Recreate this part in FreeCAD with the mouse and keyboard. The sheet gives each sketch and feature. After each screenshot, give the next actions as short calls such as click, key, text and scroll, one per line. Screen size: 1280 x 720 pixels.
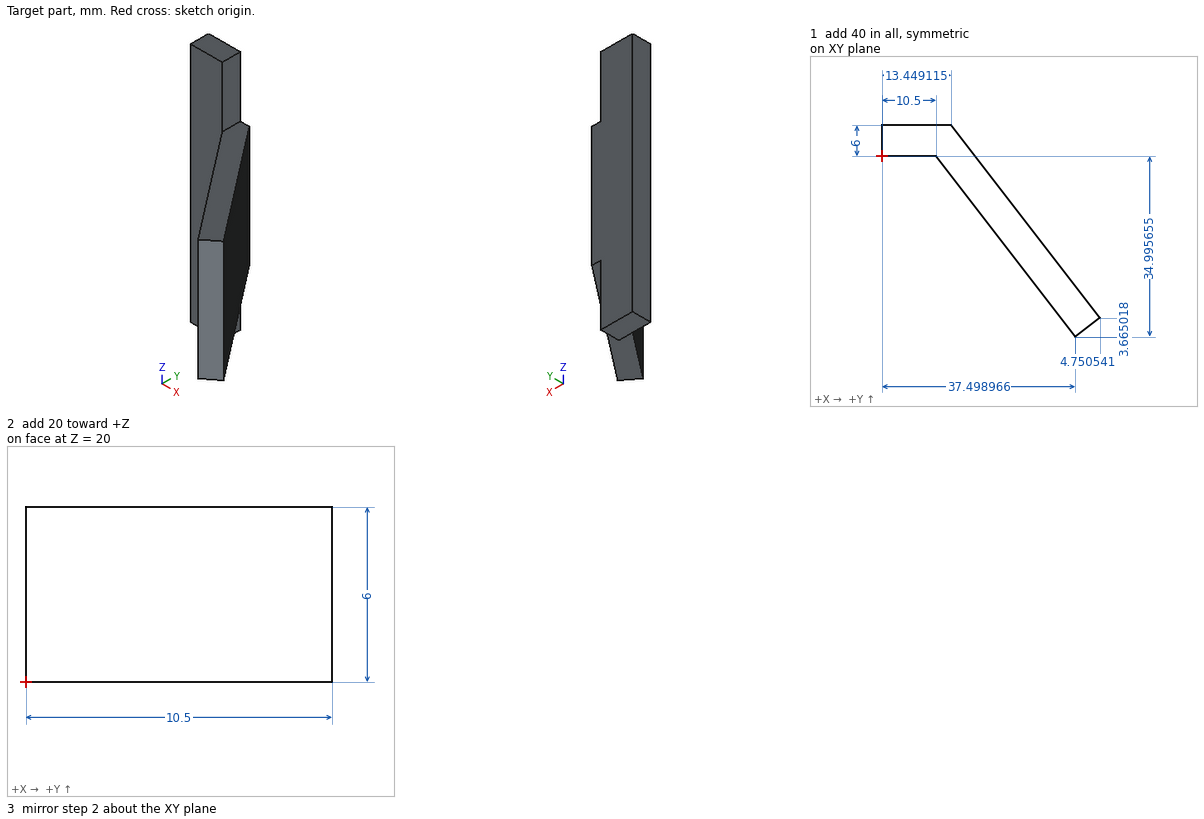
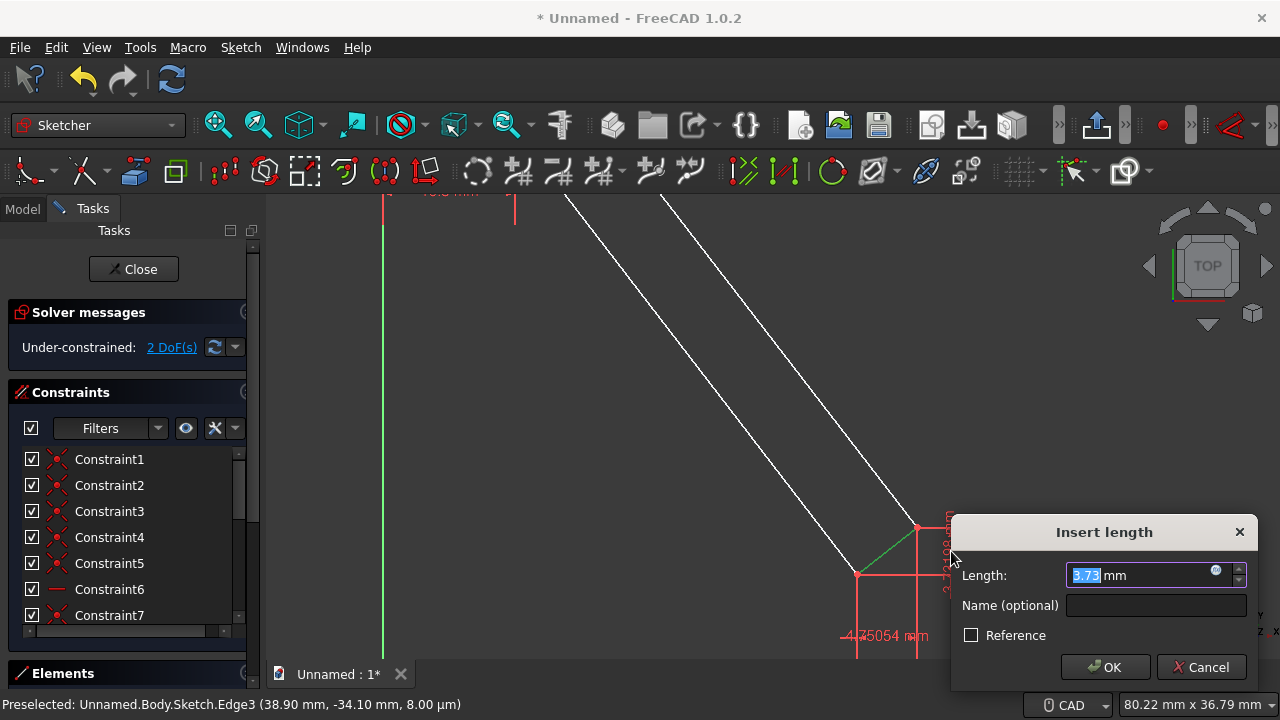
text(3.665018)
key(Return)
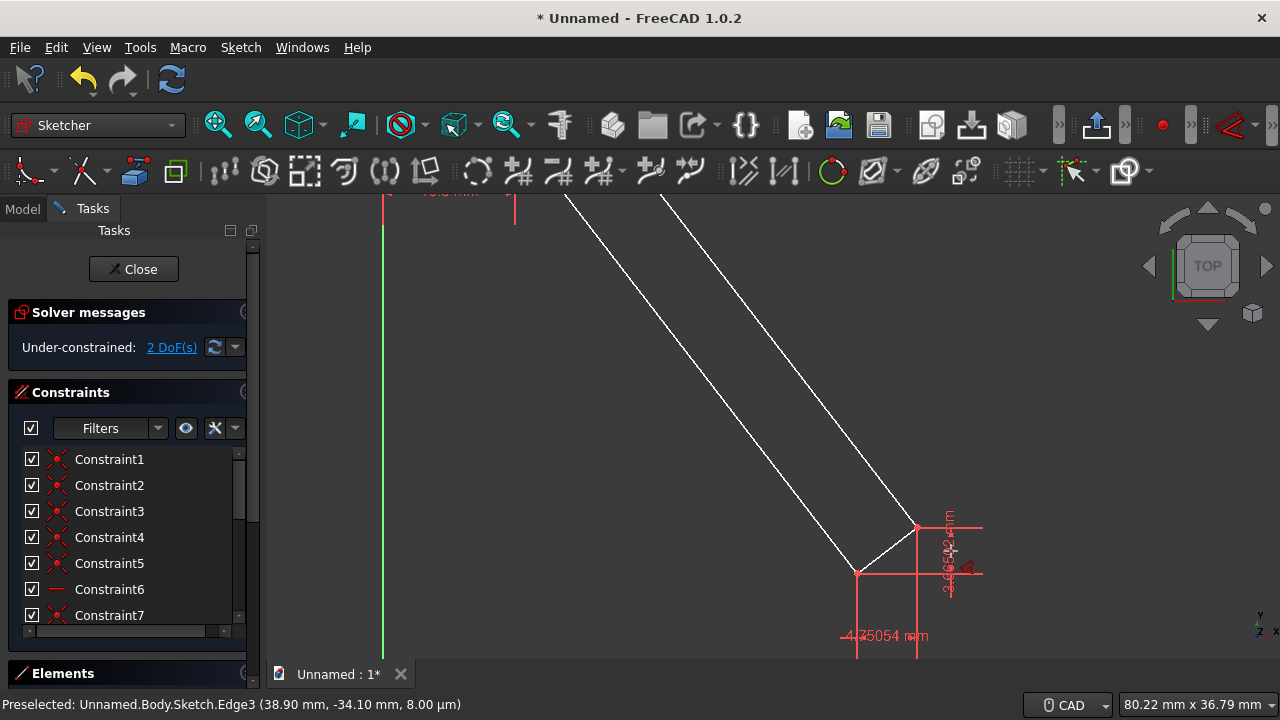
click(857, 574)
click(620, 608)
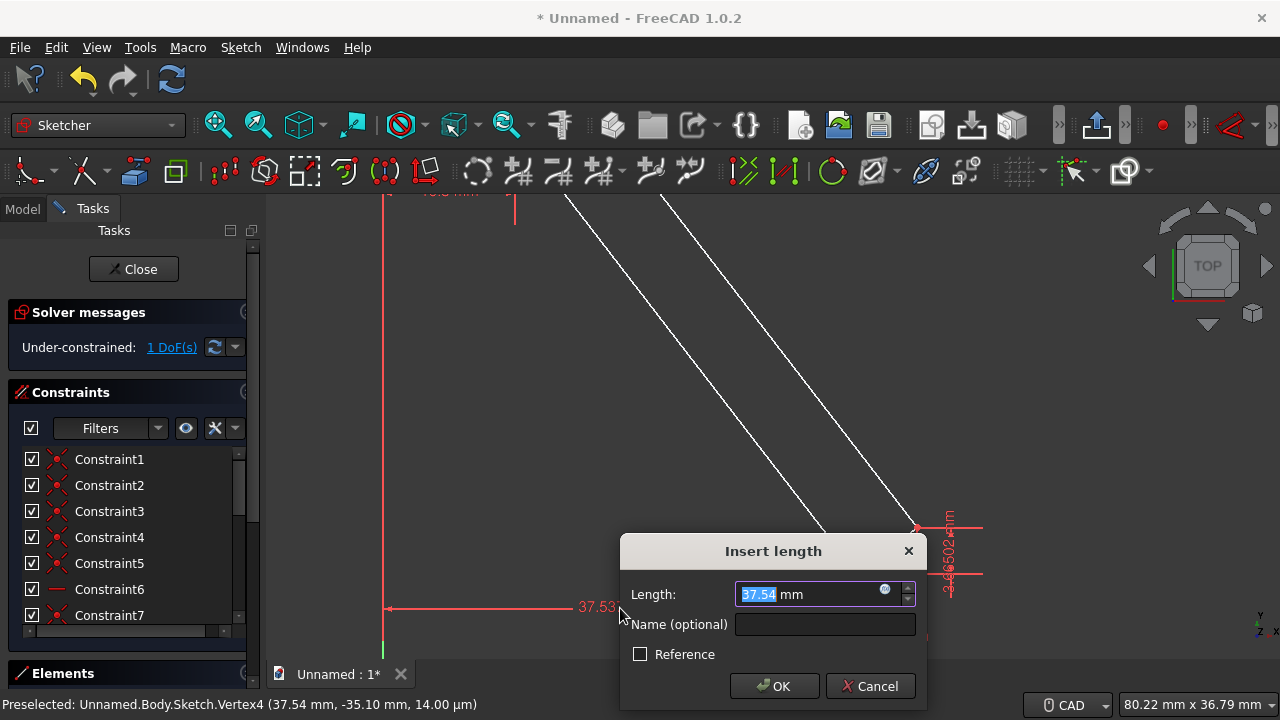
text(37.498966)
key(Return)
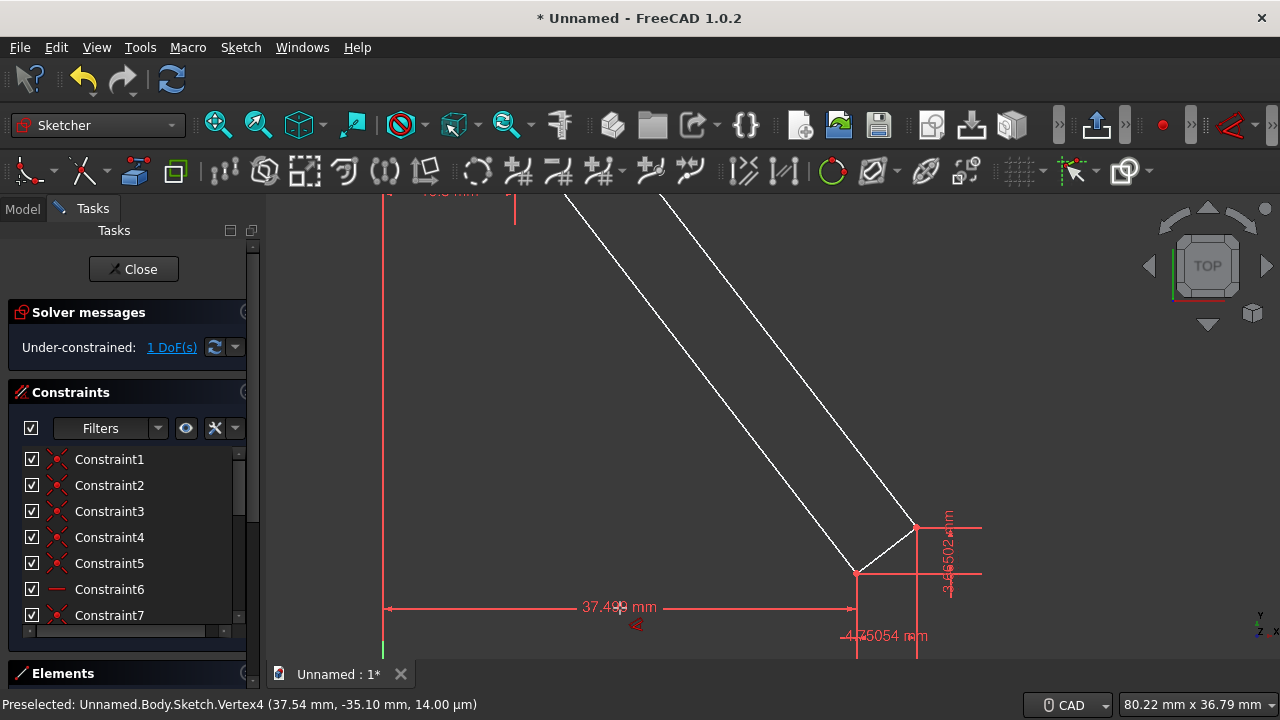
click(857, 574)
click(349, 398)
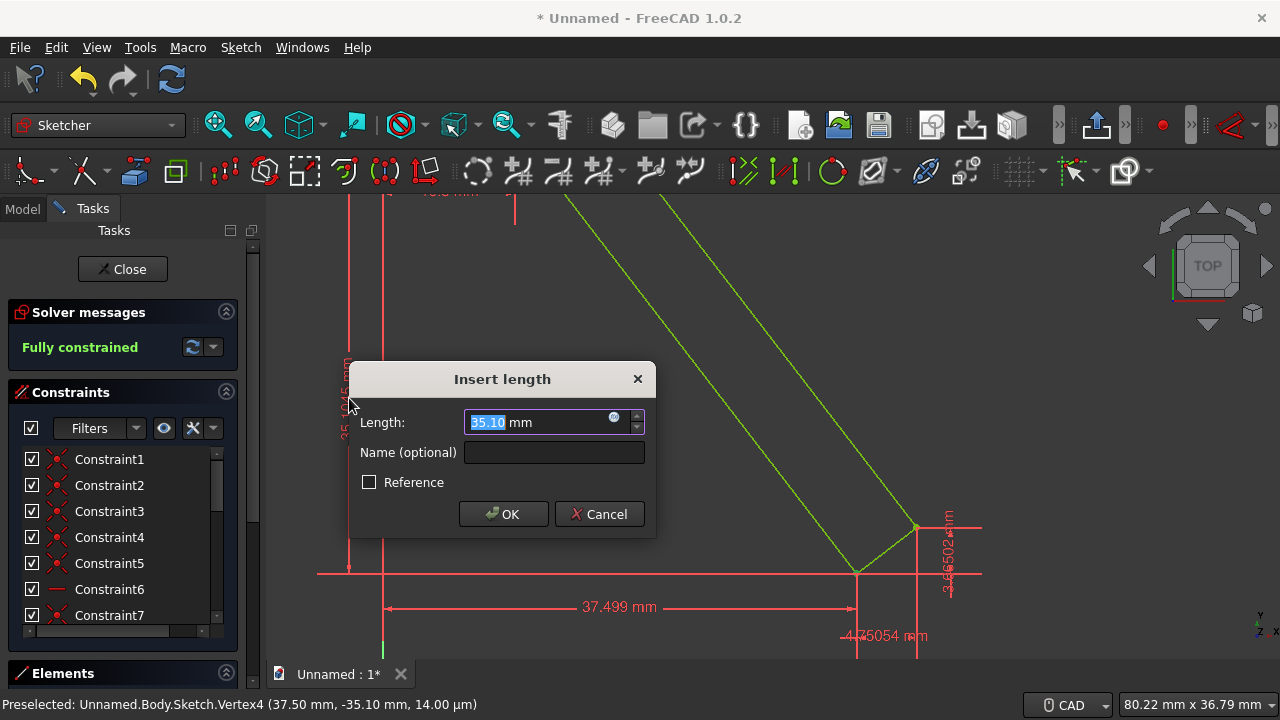
text(34.995655)
key(Return)
key(Escape)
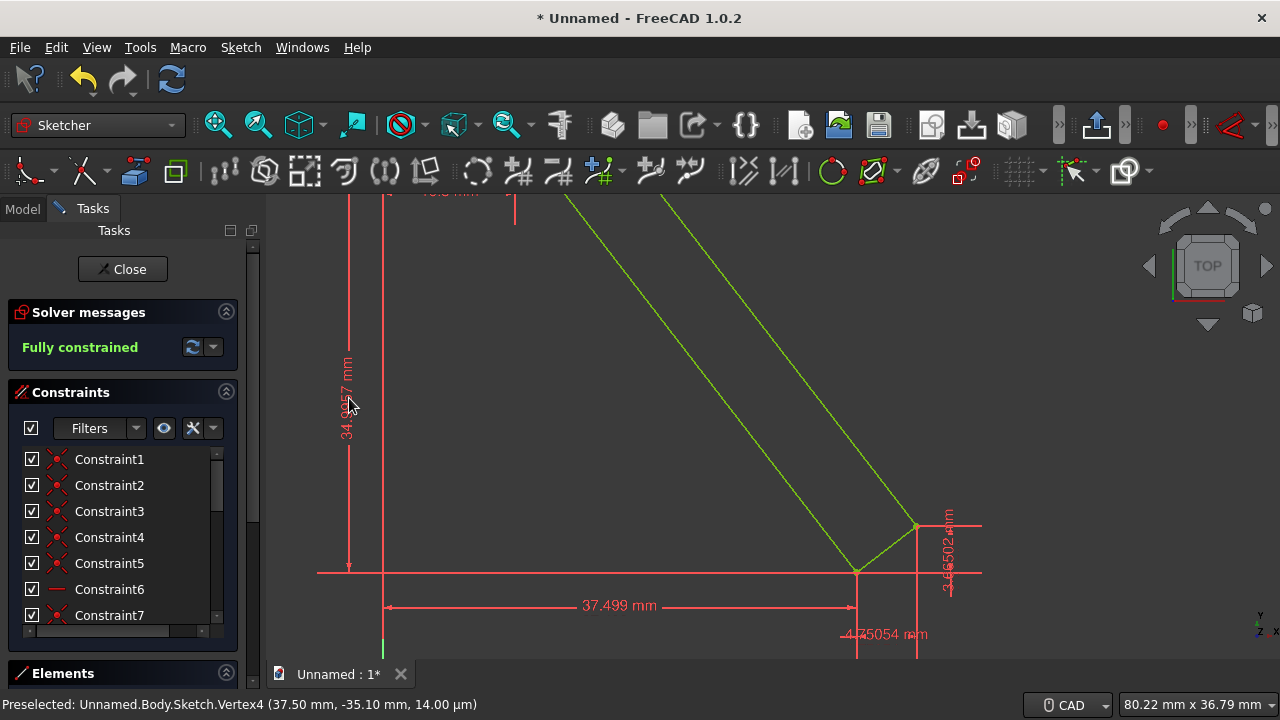
click(123, 269)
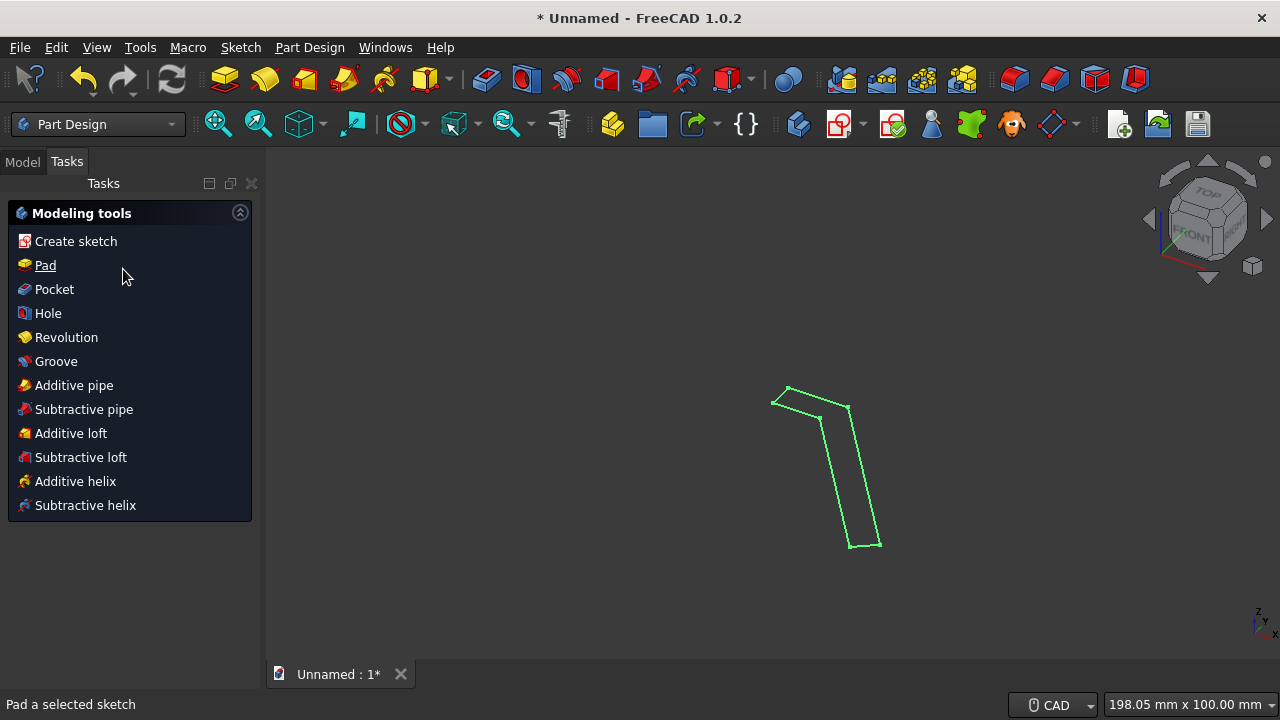
click(226, 80)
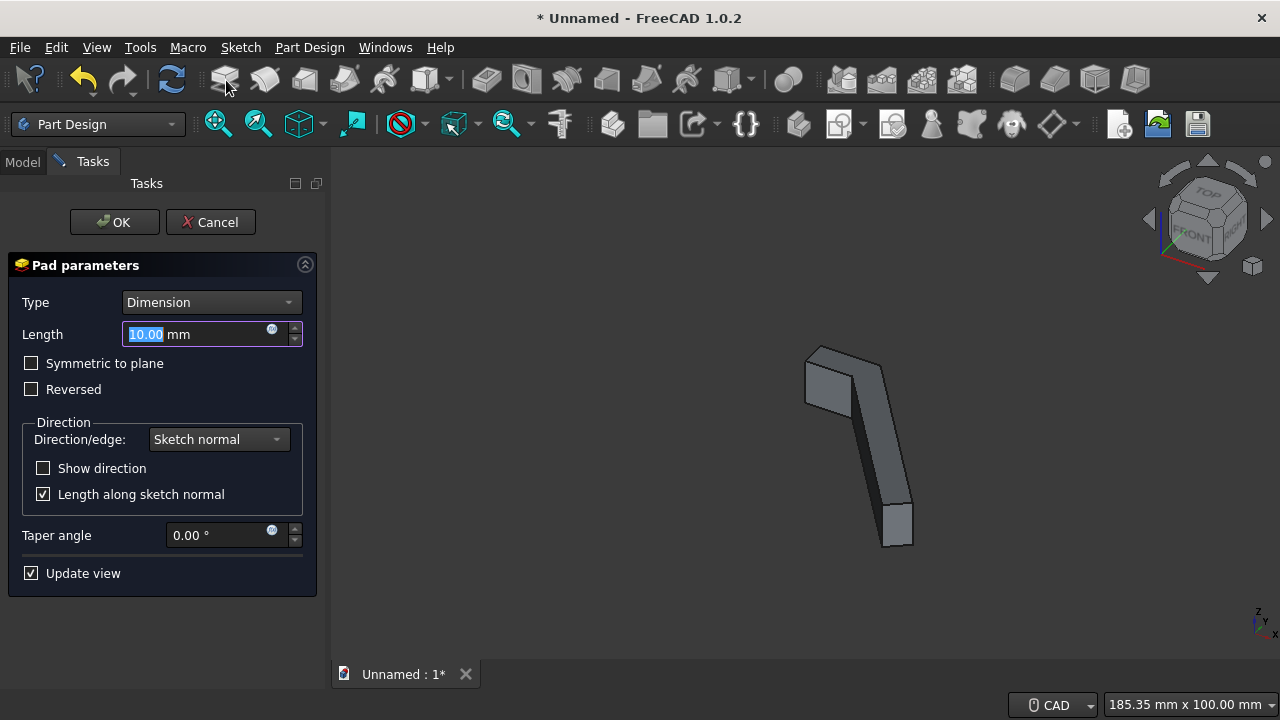
text(40)
key(Tab)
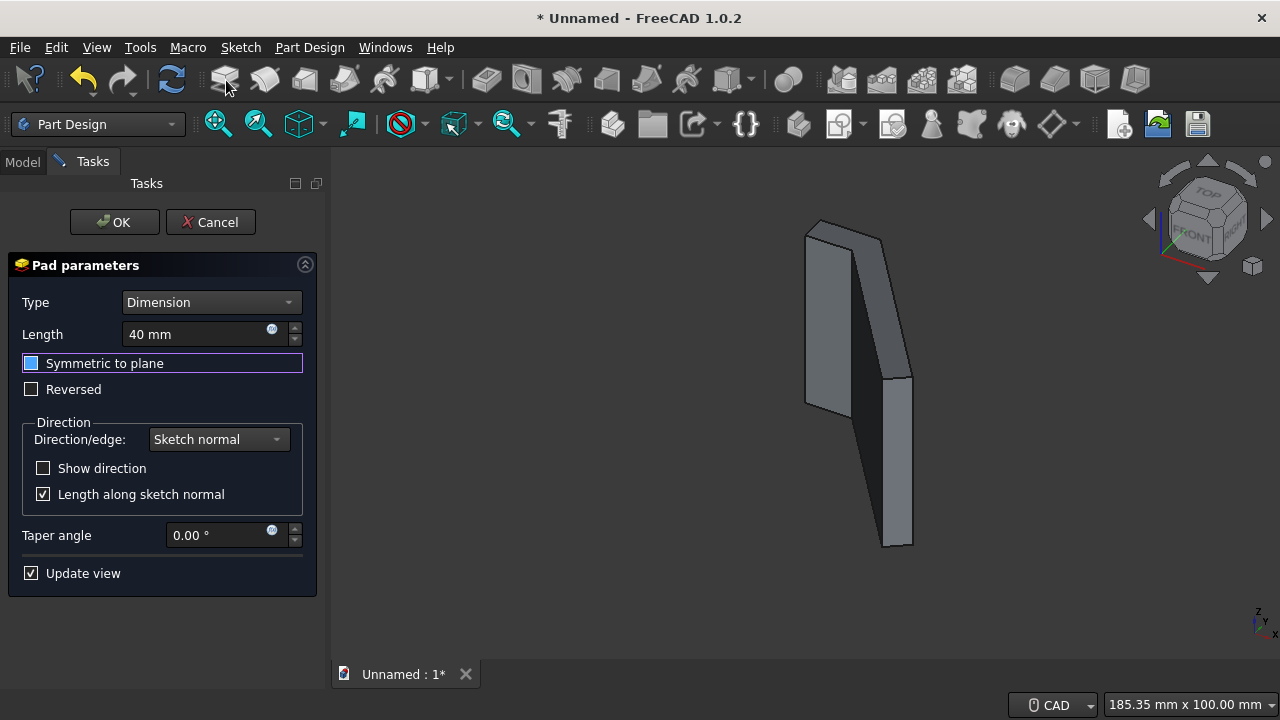
click(30, 363)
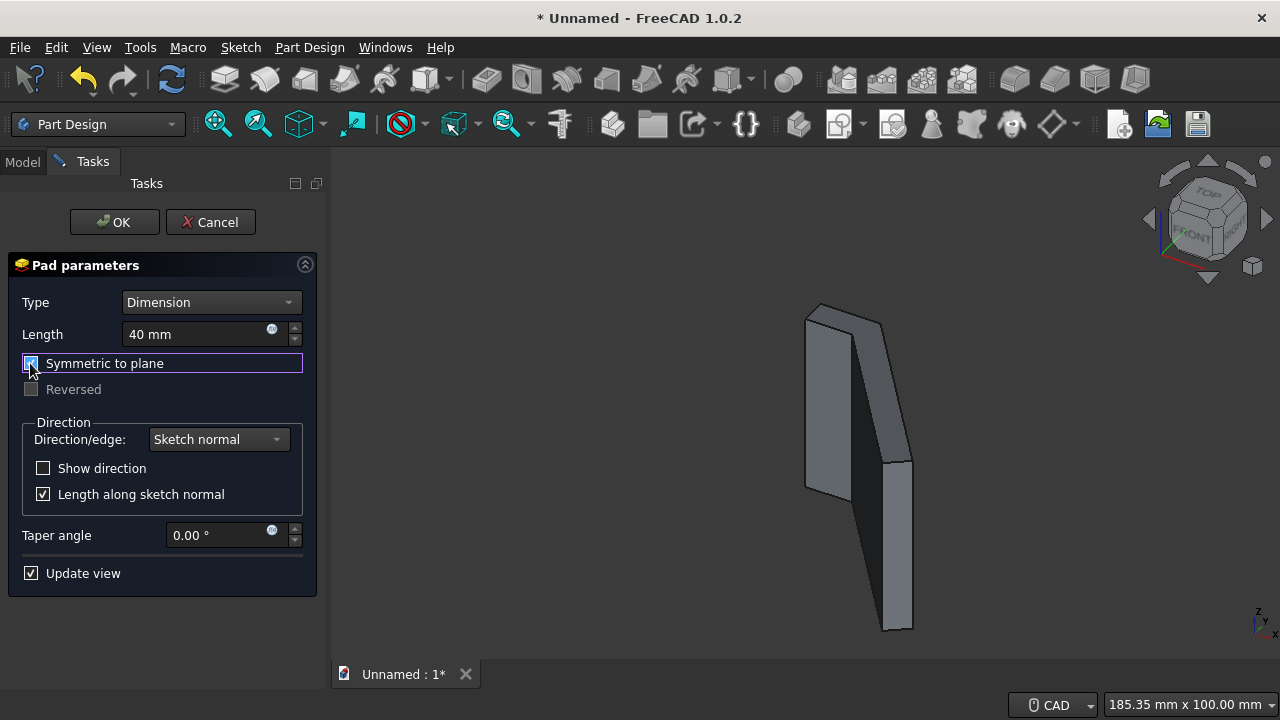
click(115, 222)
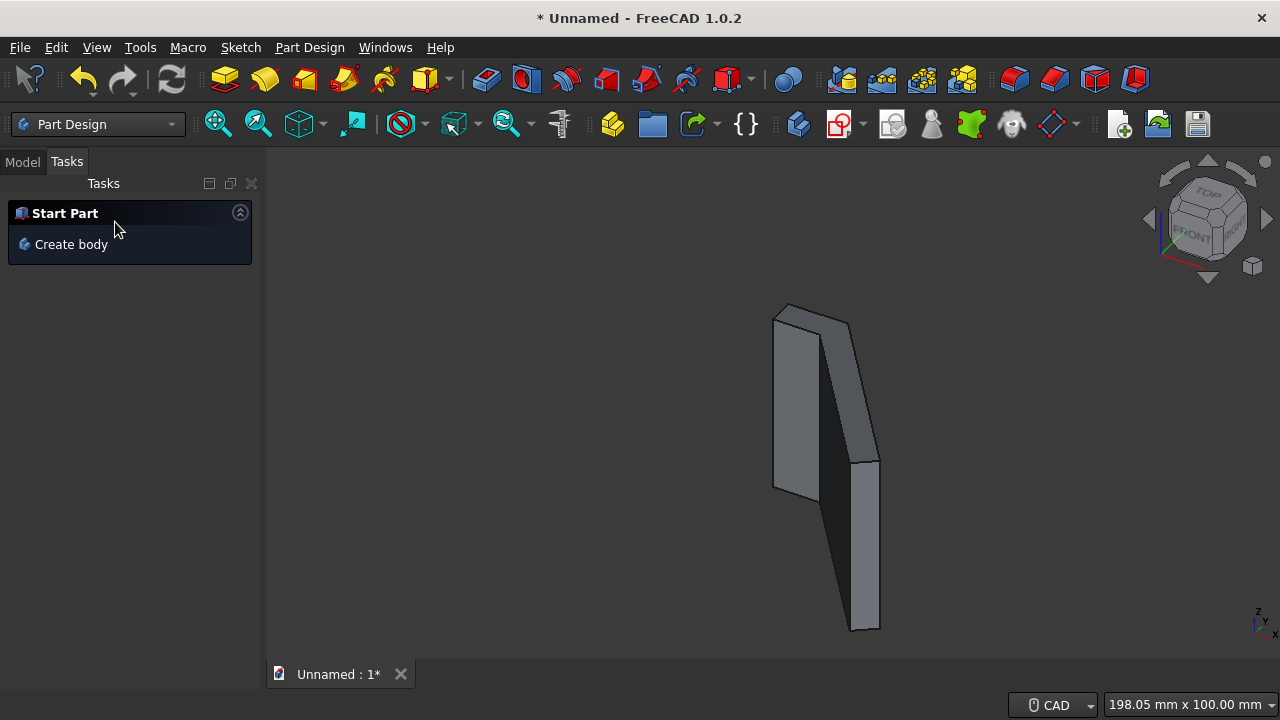
click(821, 324)